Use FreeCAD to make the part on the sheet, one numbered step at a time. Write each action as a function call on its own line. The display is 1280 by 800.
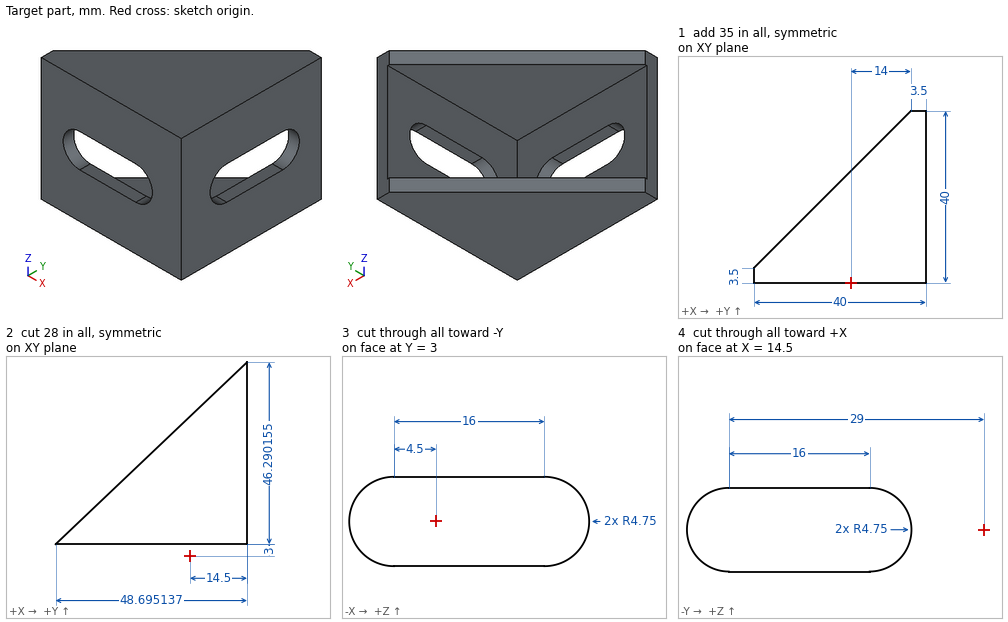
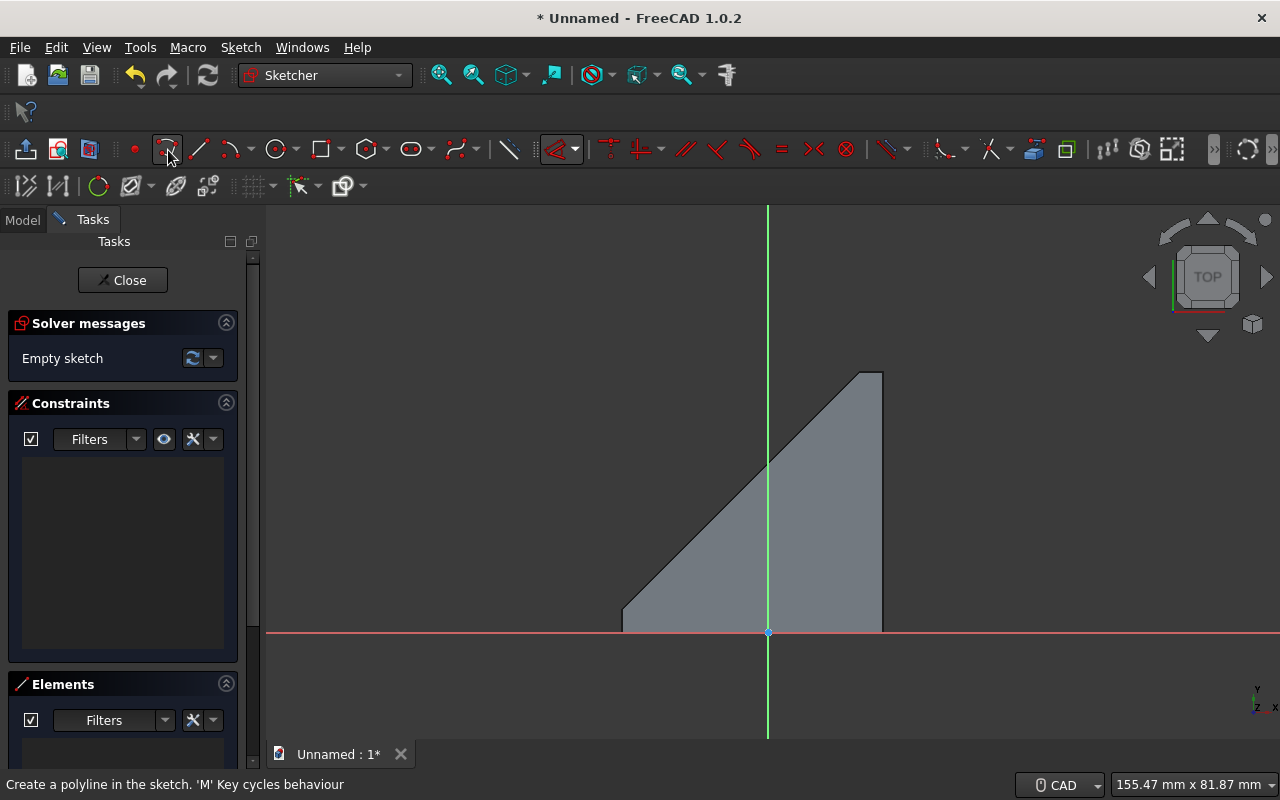
click(863, 613)
click(863, 311)
click(545, 613)
click(863, 614)
key(Escape)
key(Escape)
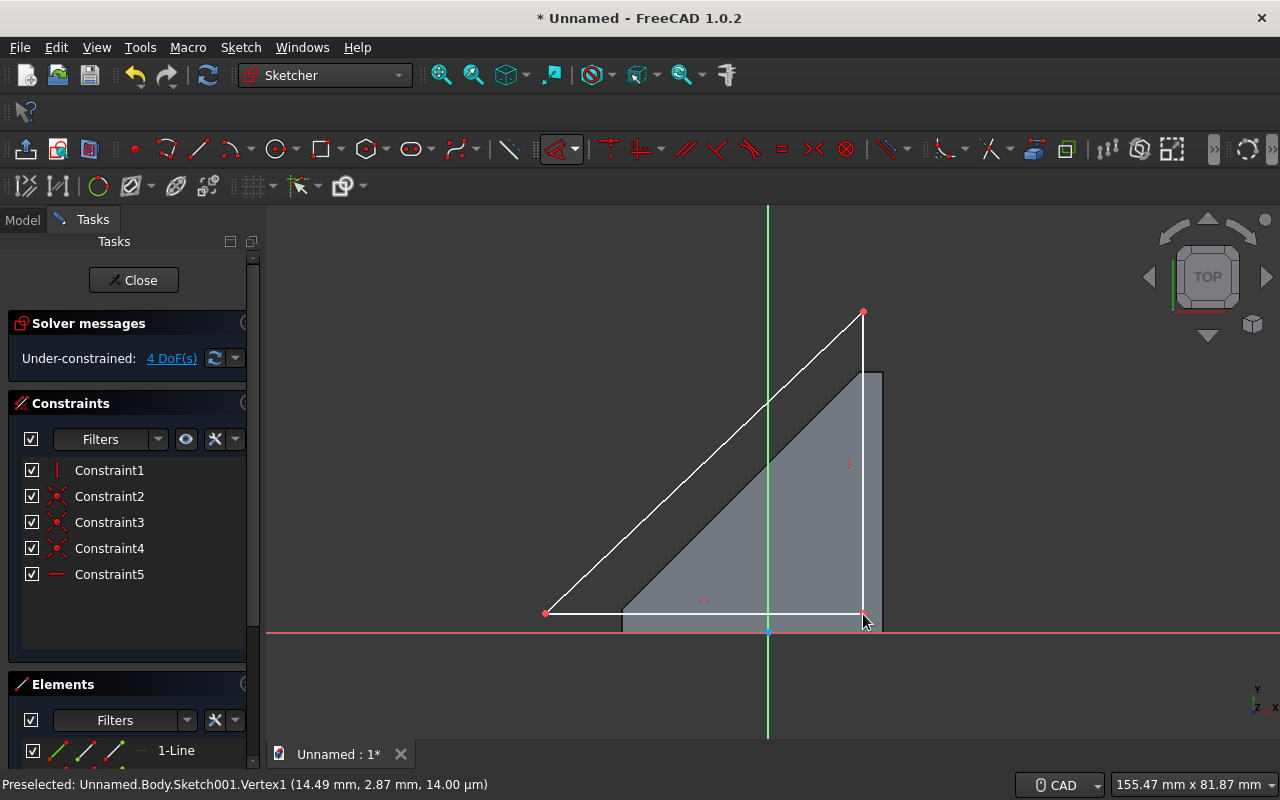
scroll(863, 614, up, 4)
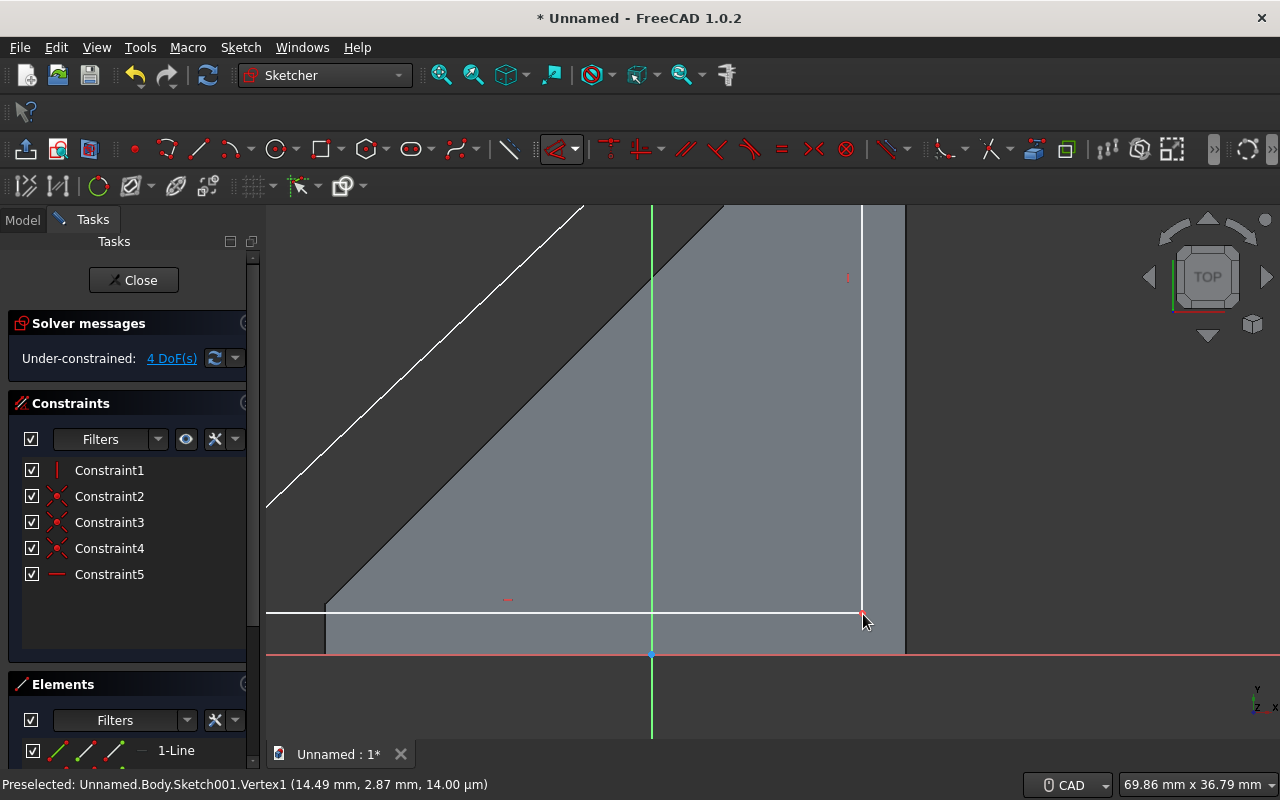
click(862, 613)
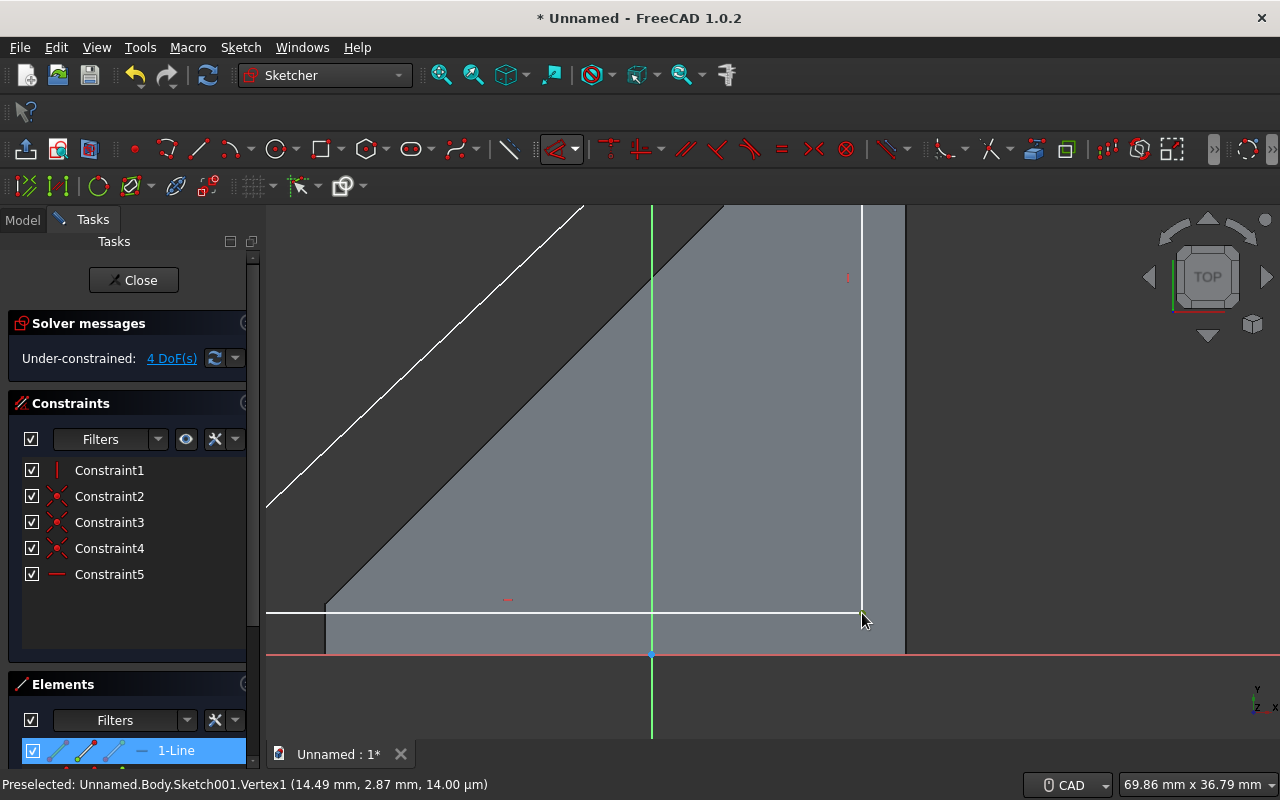
key(i)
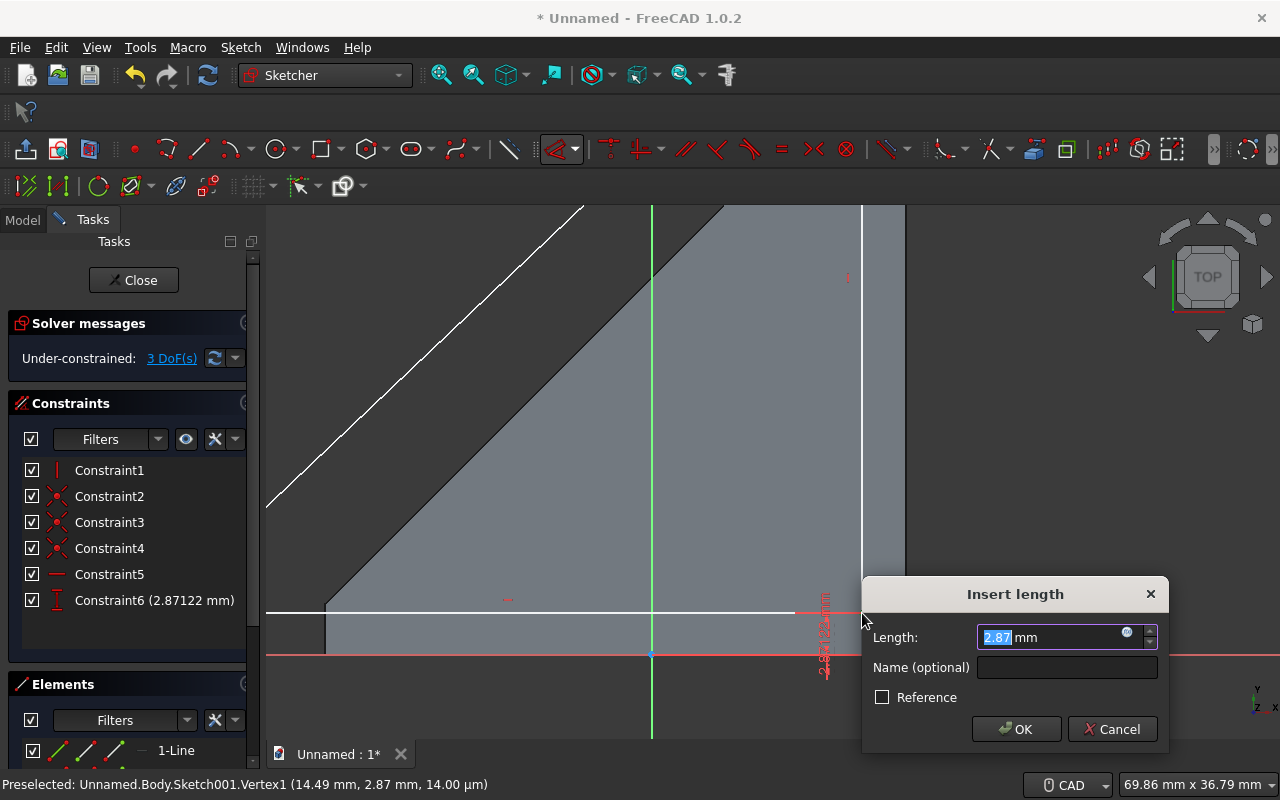
text(3)
key(Return)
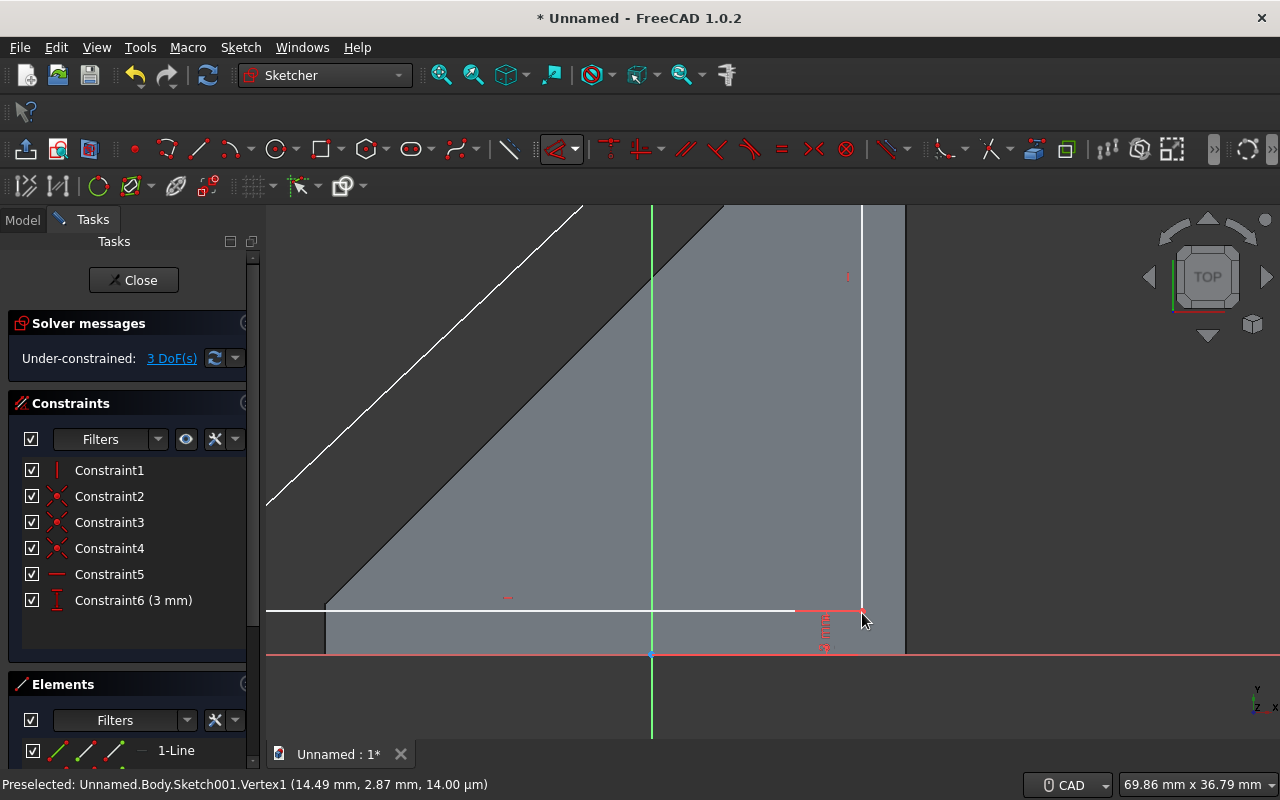
click(862, 611)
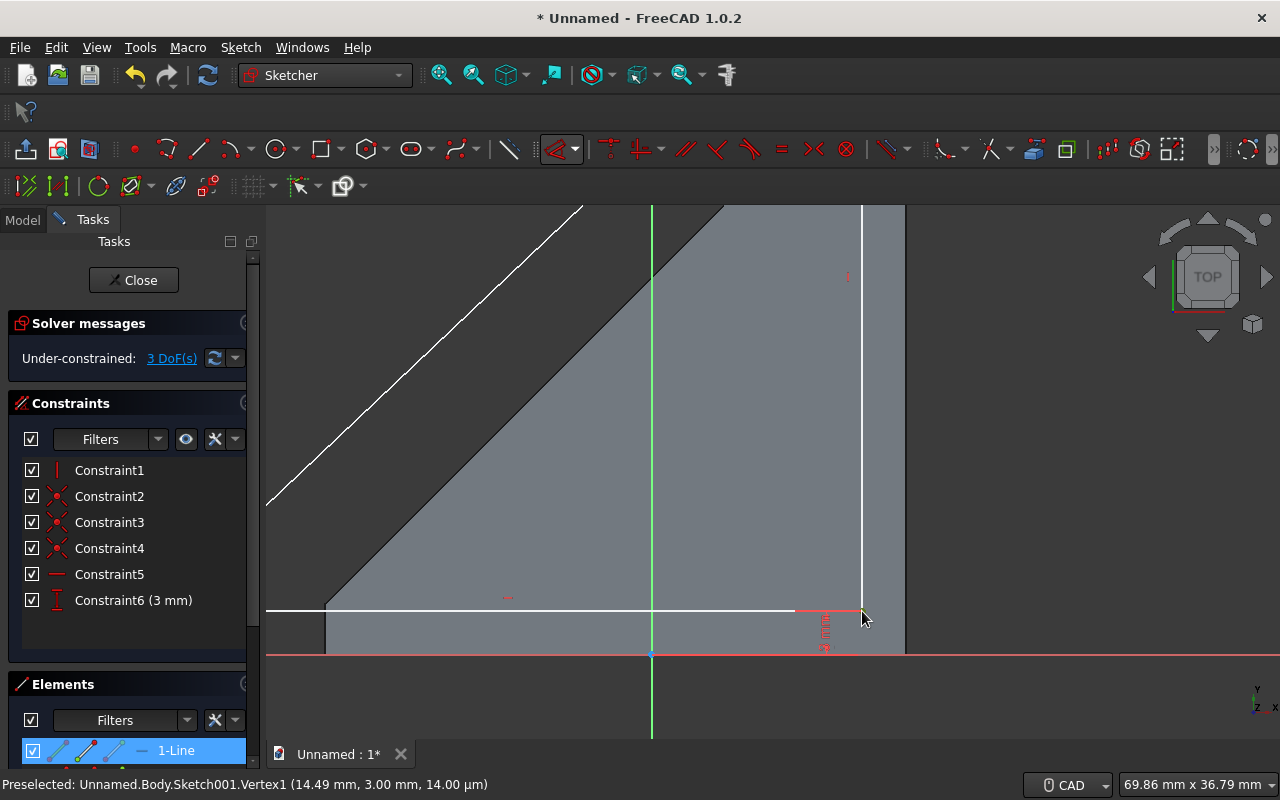
click(578, 150)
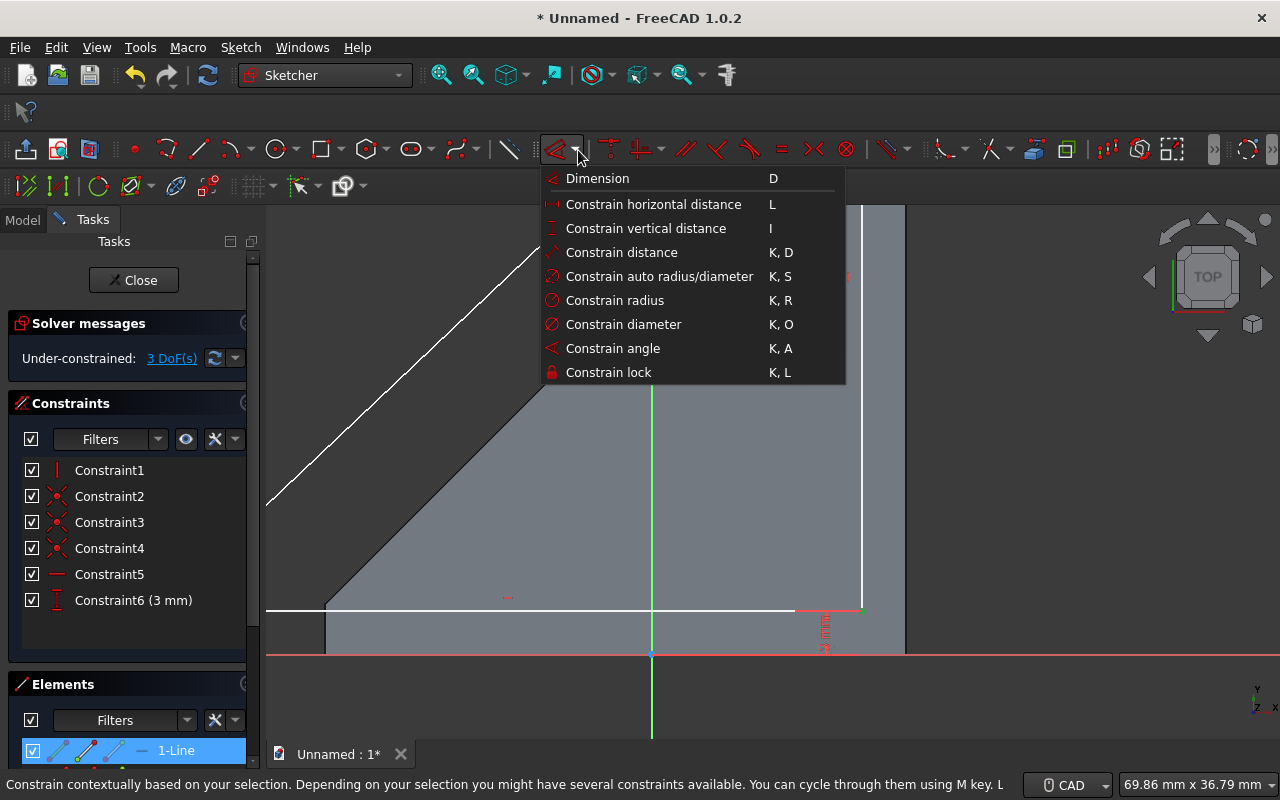
click(693, 204)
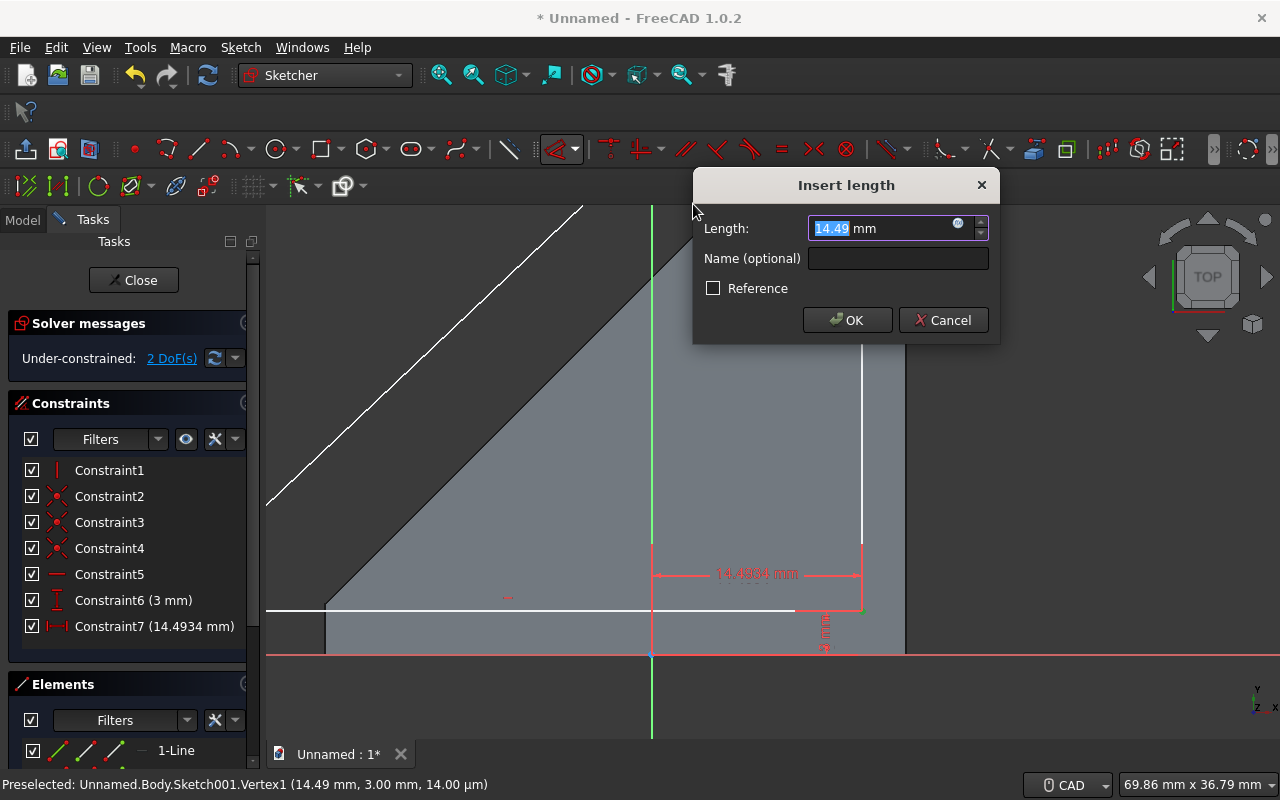
text(14.5)
key(Return)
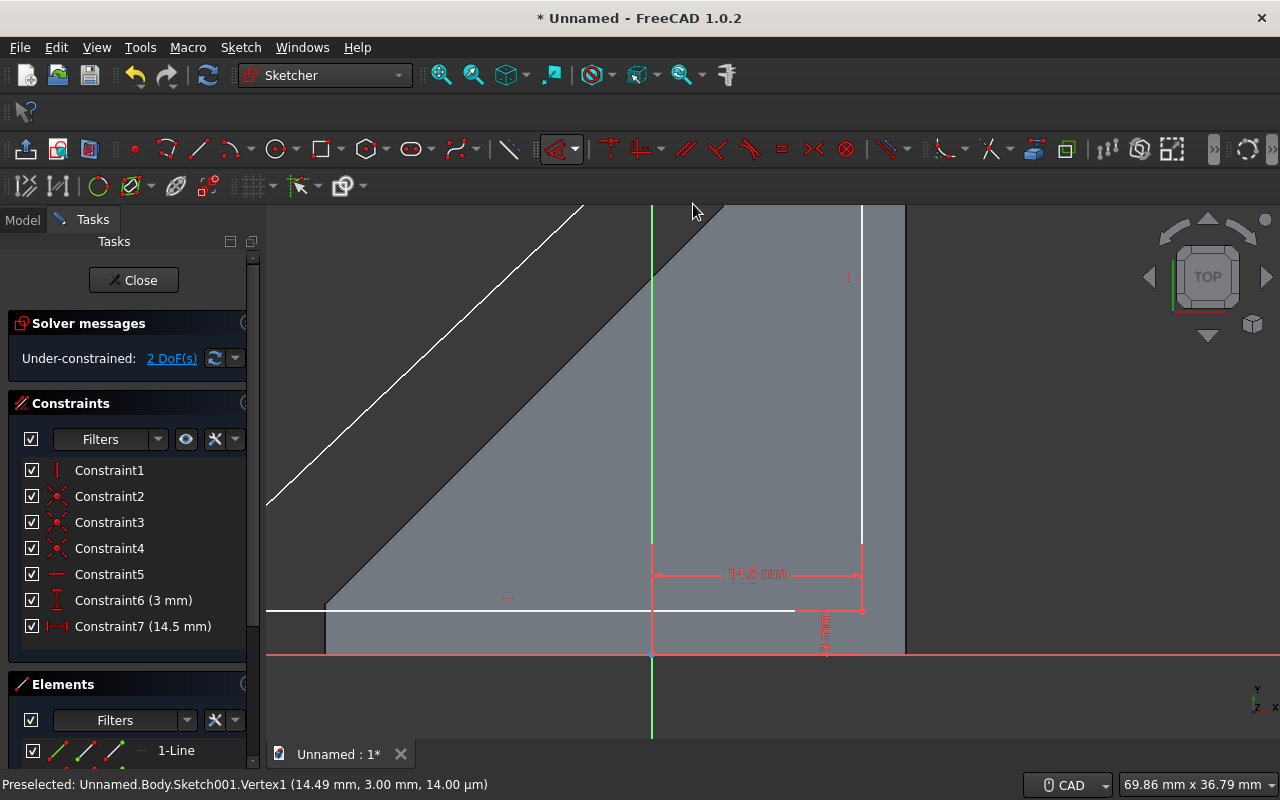
click(862, 410)